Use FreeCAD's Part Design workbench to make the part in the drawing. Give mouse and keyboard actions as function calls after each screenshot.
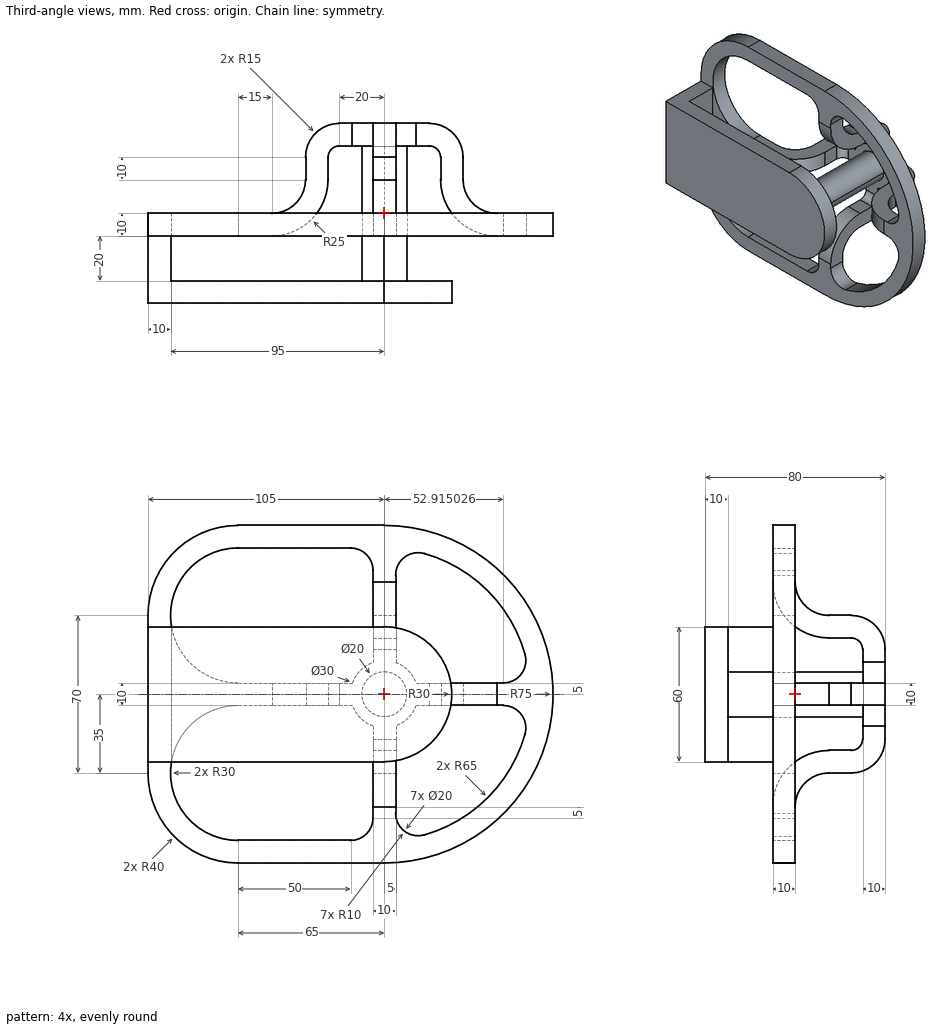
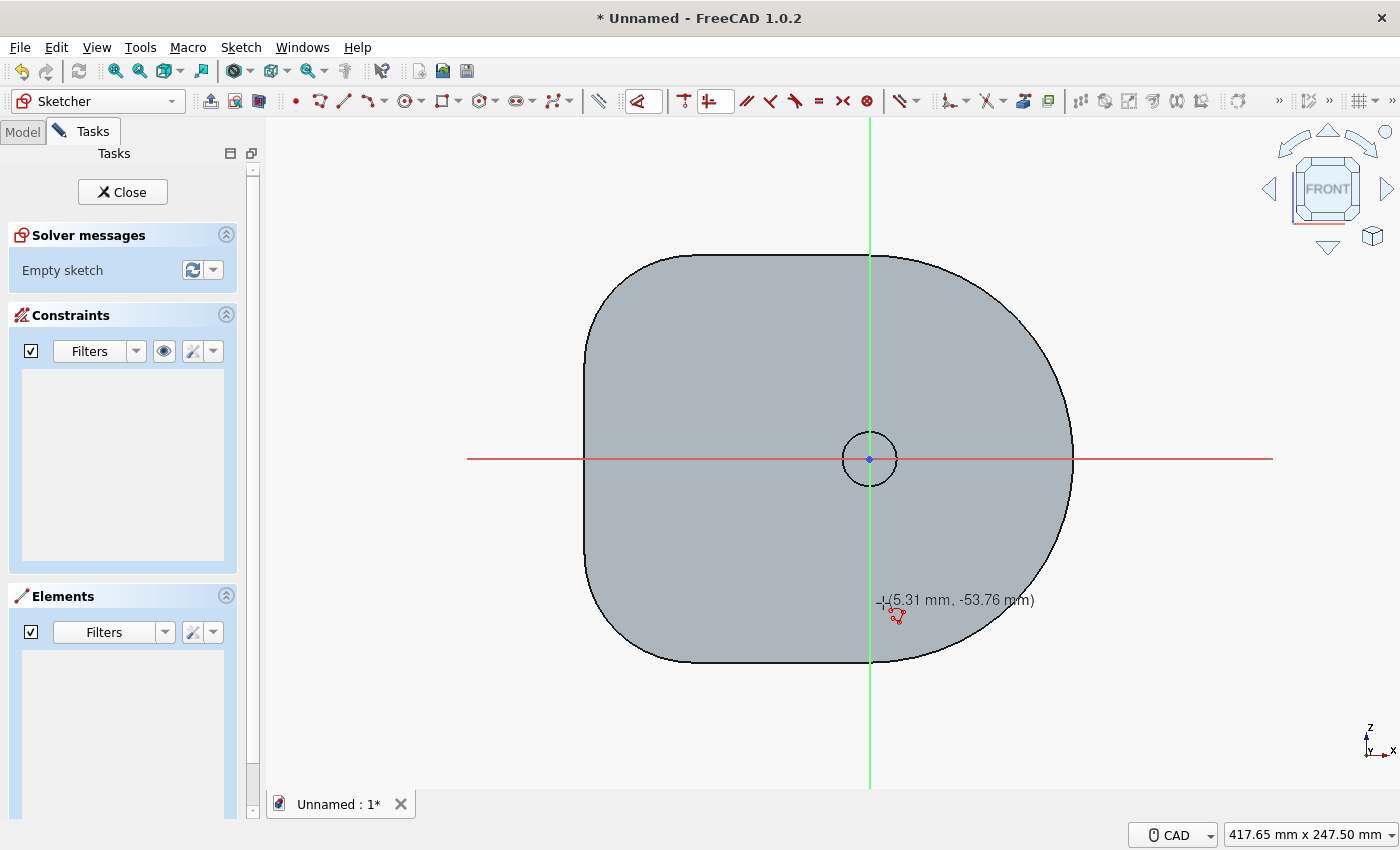
scroll(883, 595, up, 4)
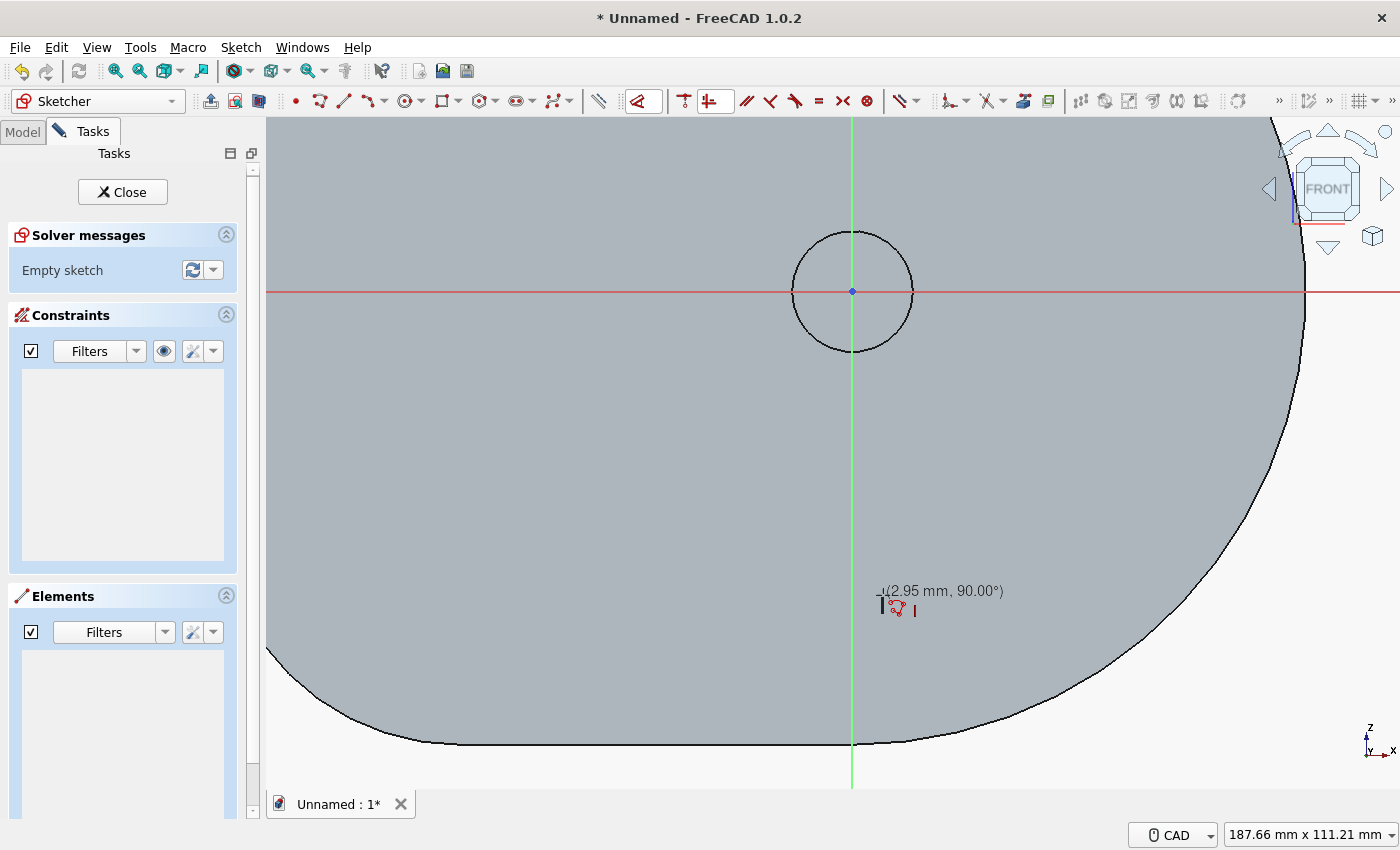
click(882, 594)
click(822, 594)
click(822, 624)
right_click(822, 624)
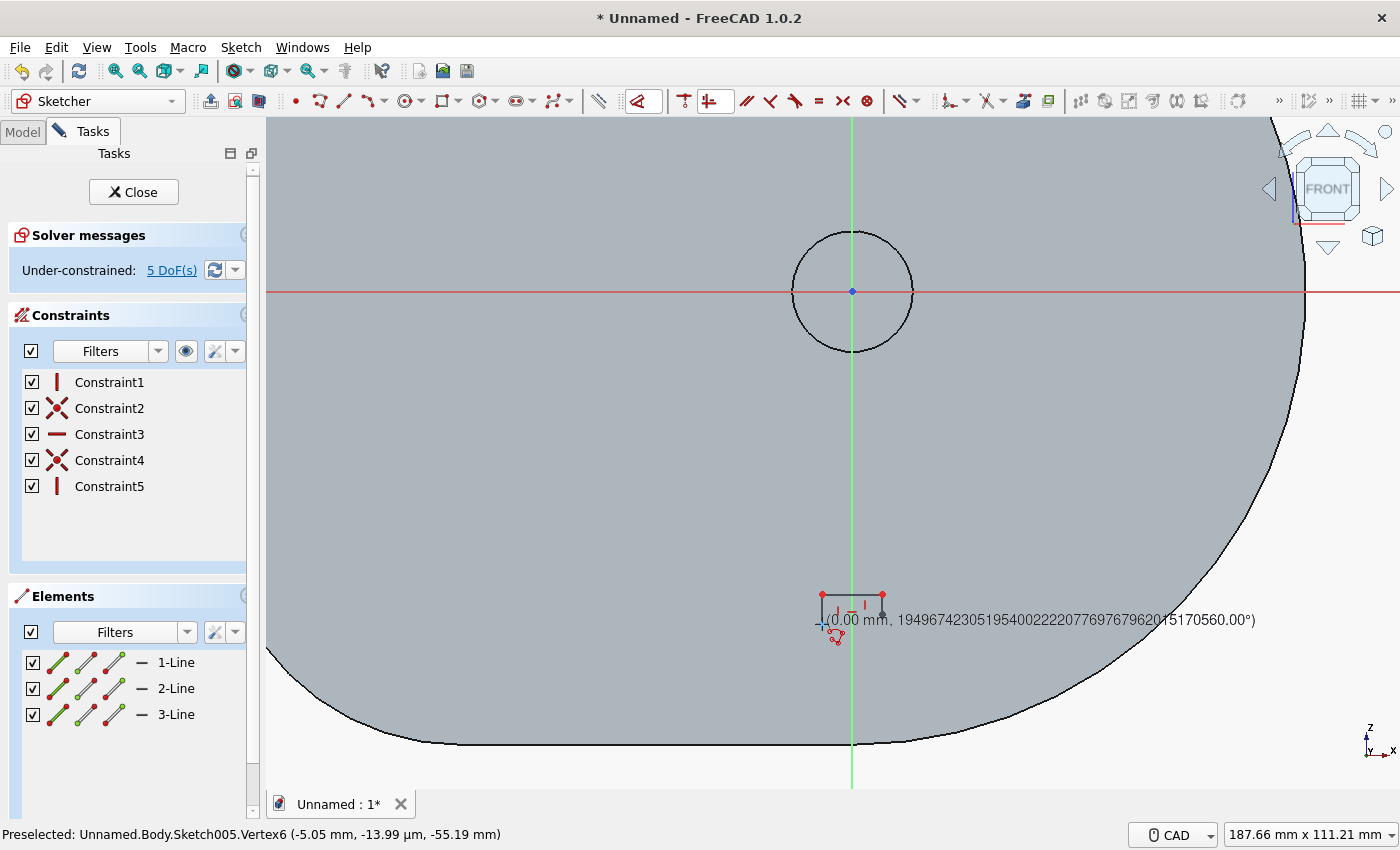
click(344, 102)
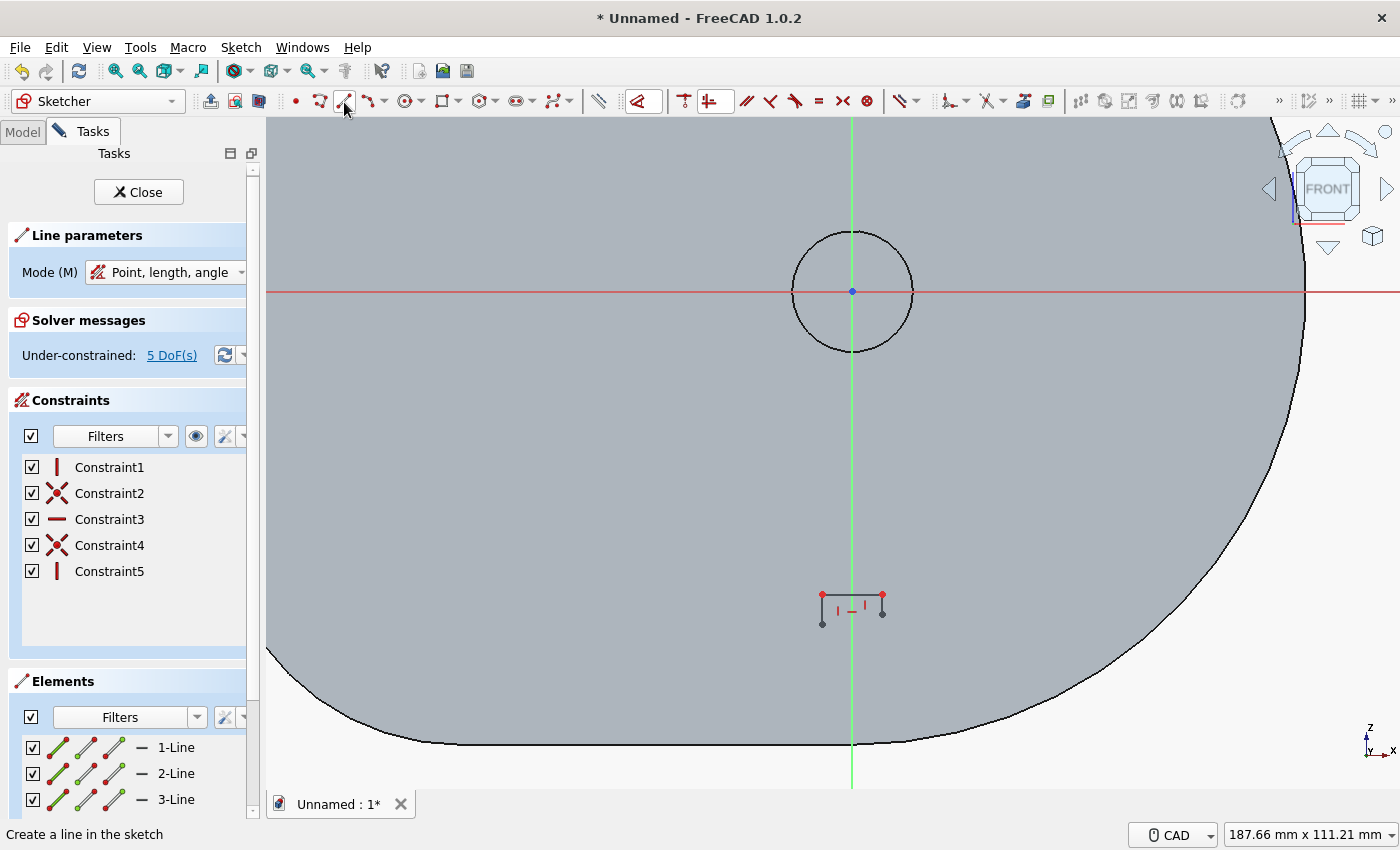
click(762, 684)
click(460, 684)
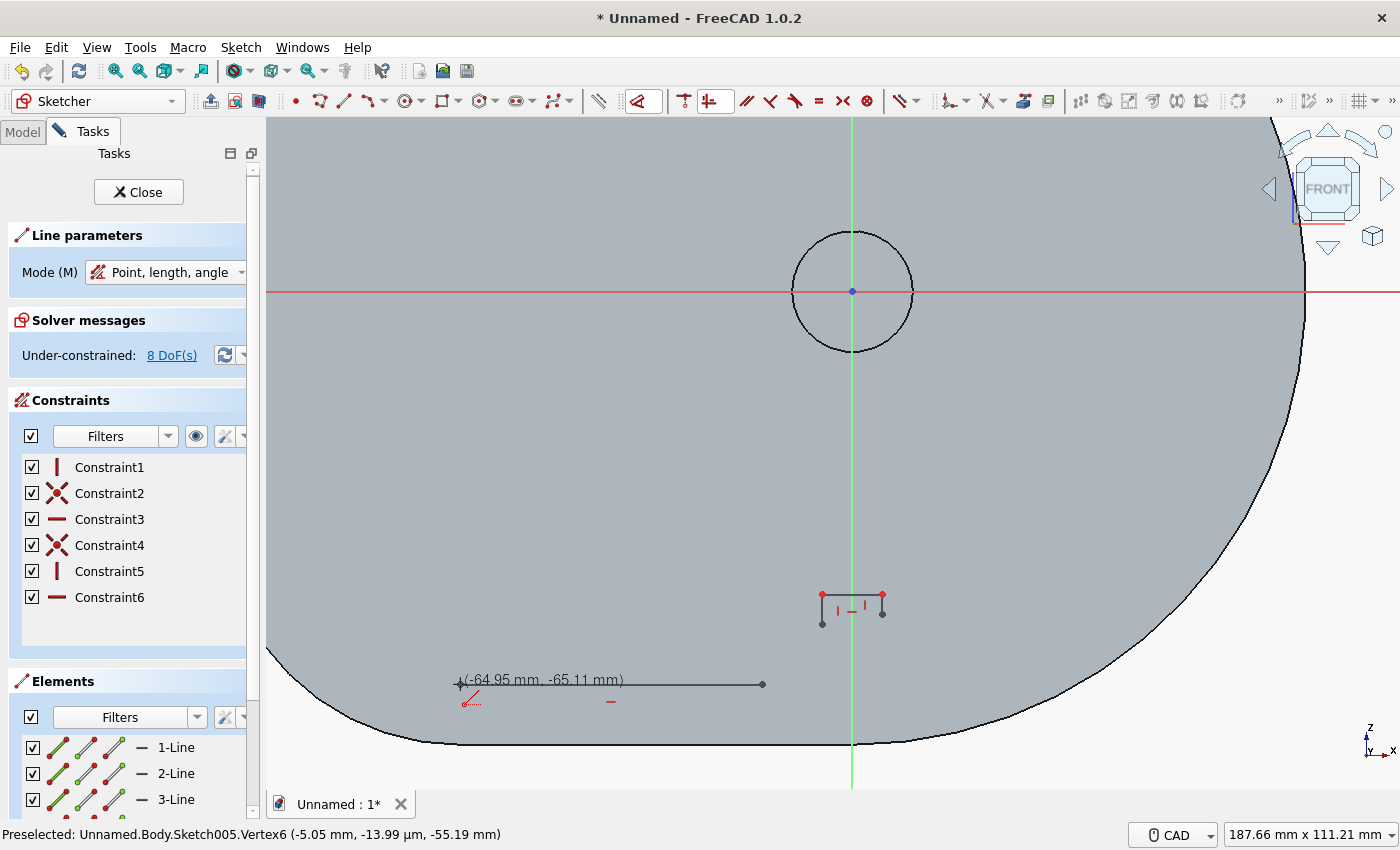
click(460, 322)
click(460, 261)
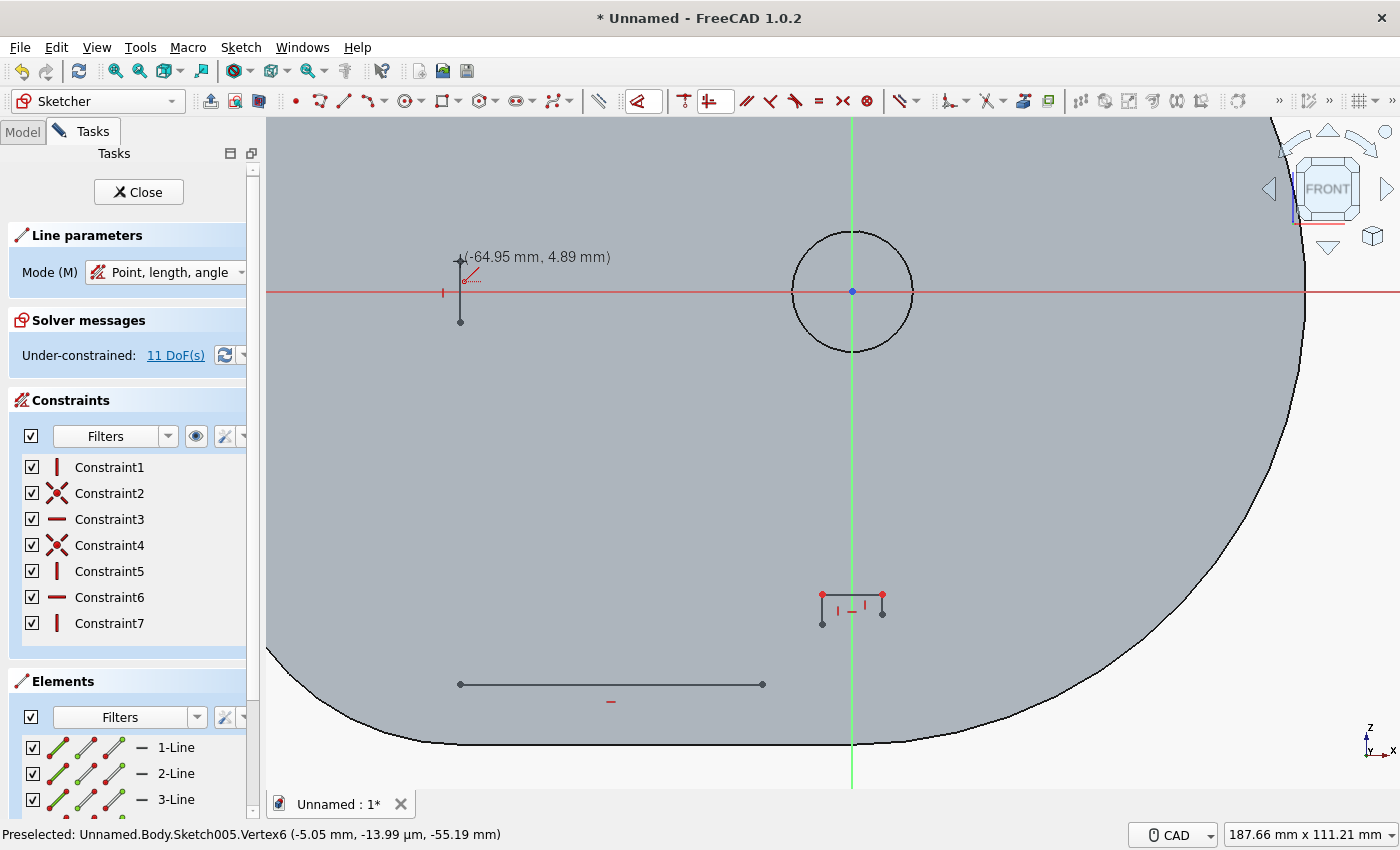
scroll(777, 649, down, 3)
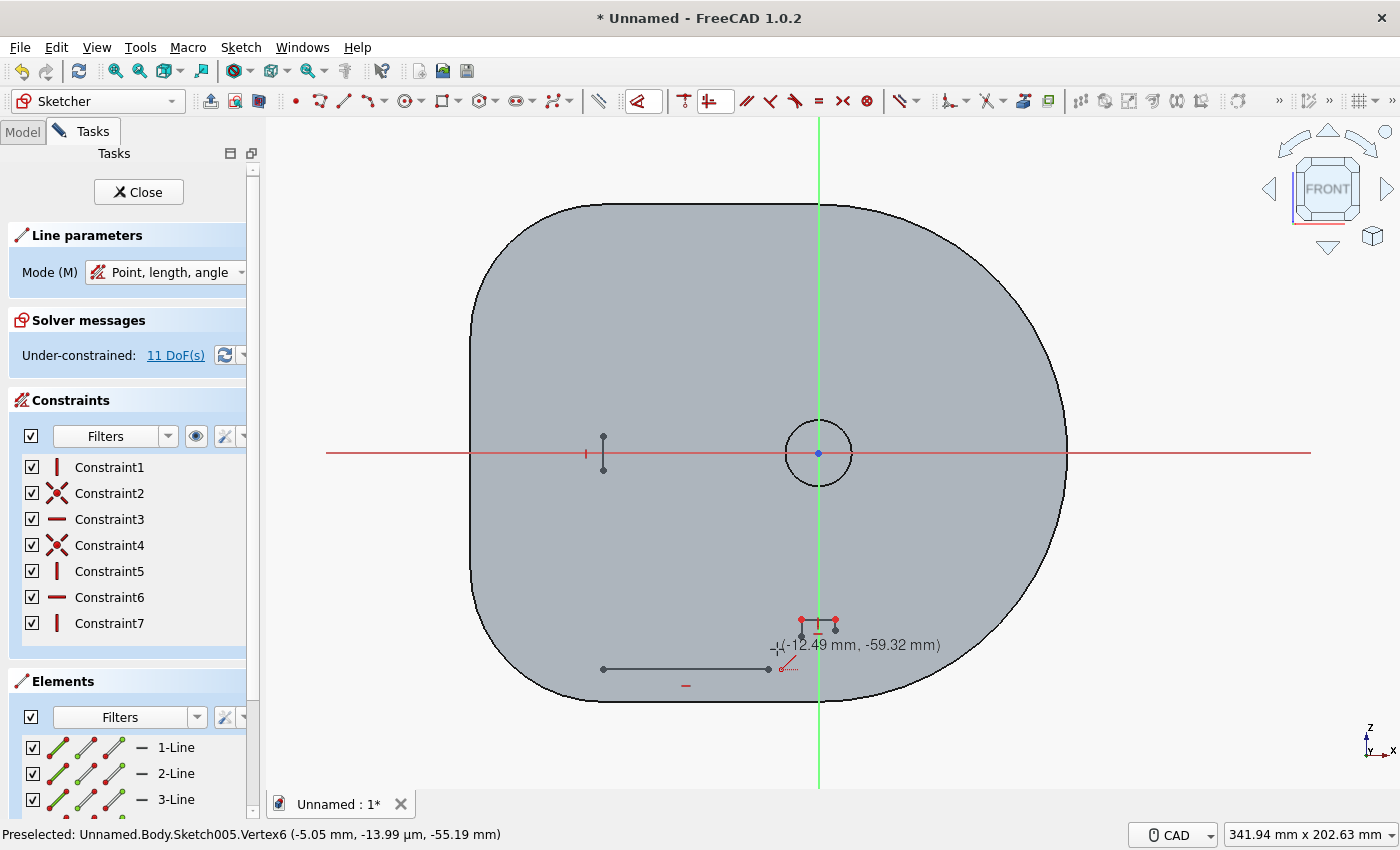
click(603, 238)
click(769, 238)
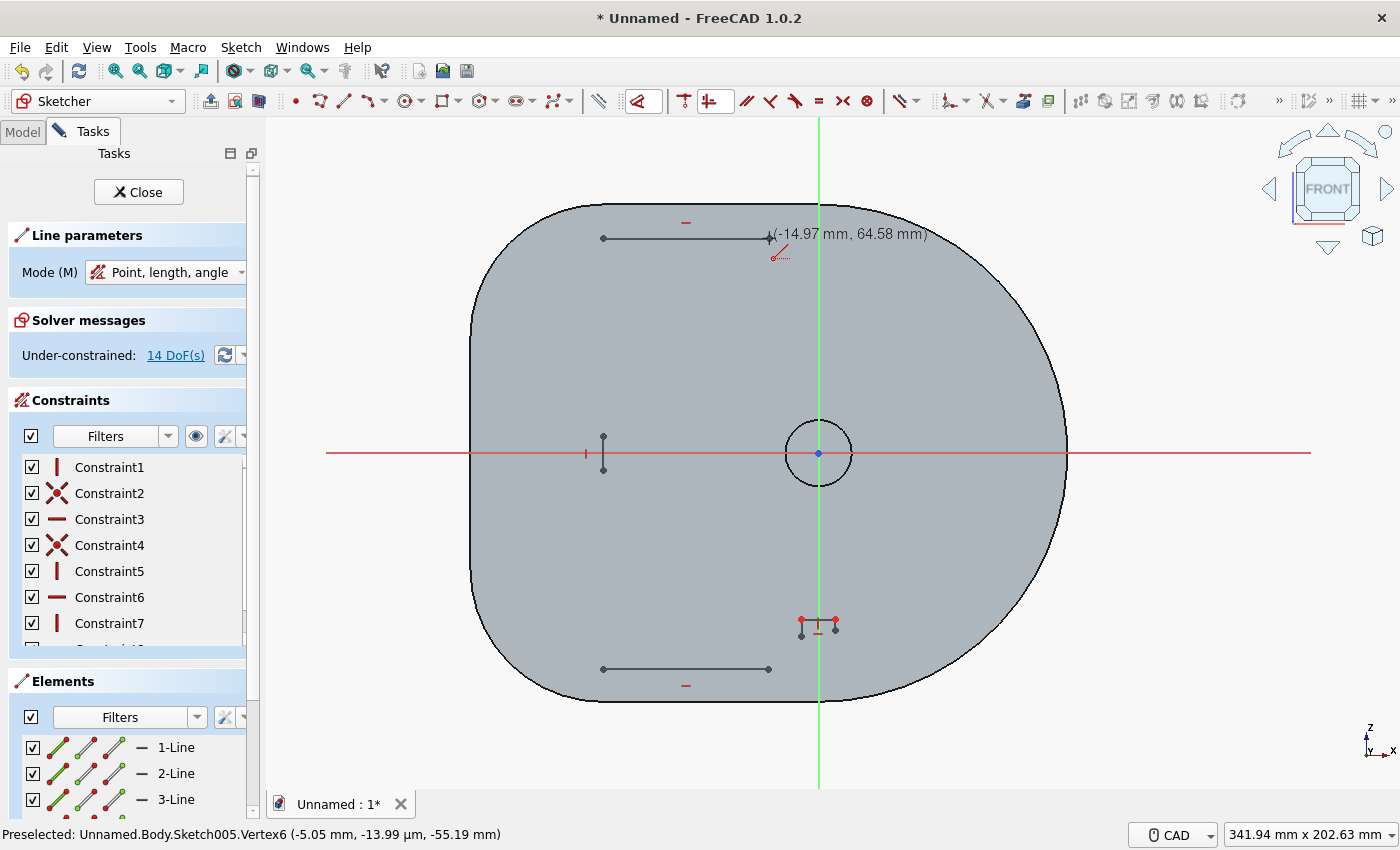
click(320, 102)